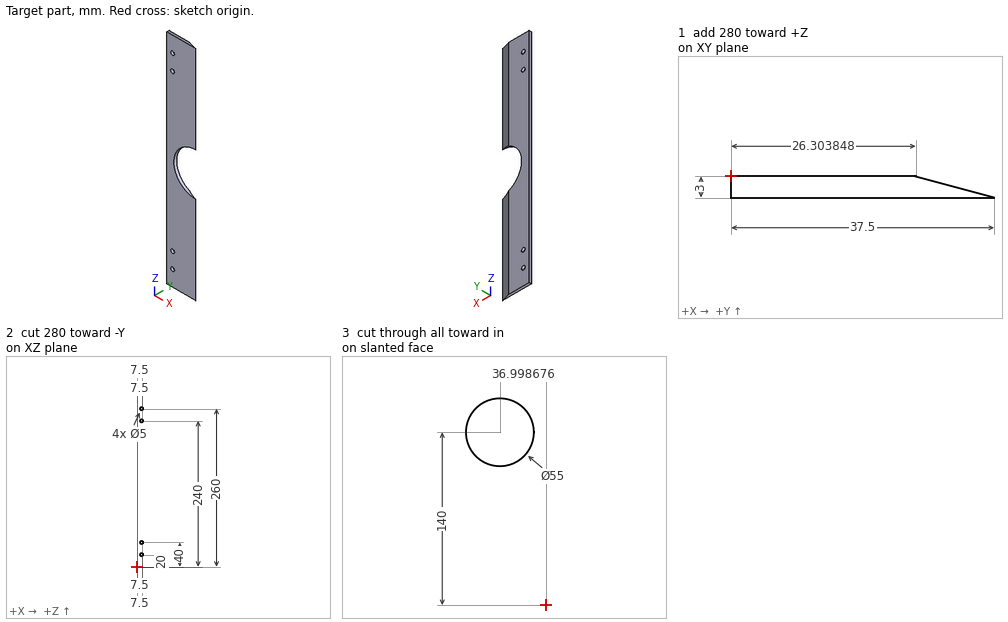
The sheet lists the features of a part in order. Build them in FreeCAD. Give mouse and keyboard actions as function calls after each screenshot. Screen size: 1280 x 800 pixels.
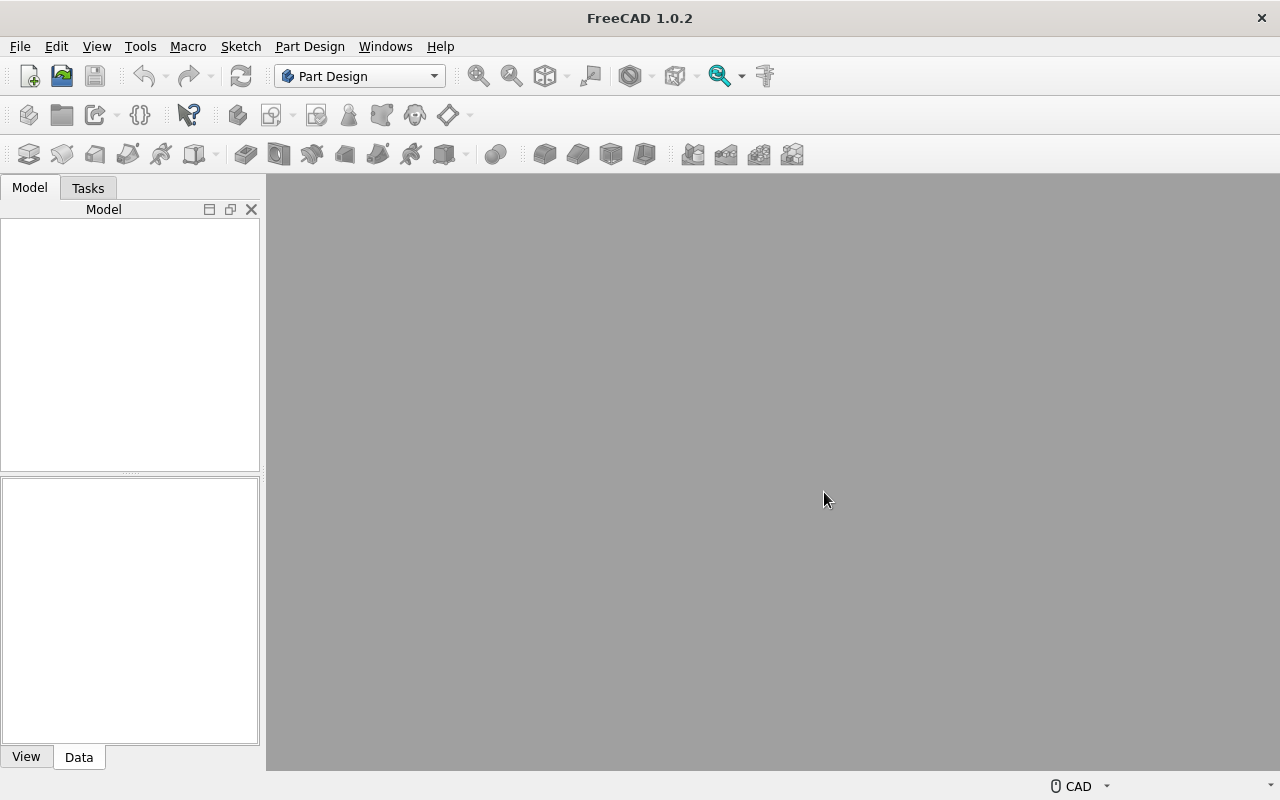
click(29, 76)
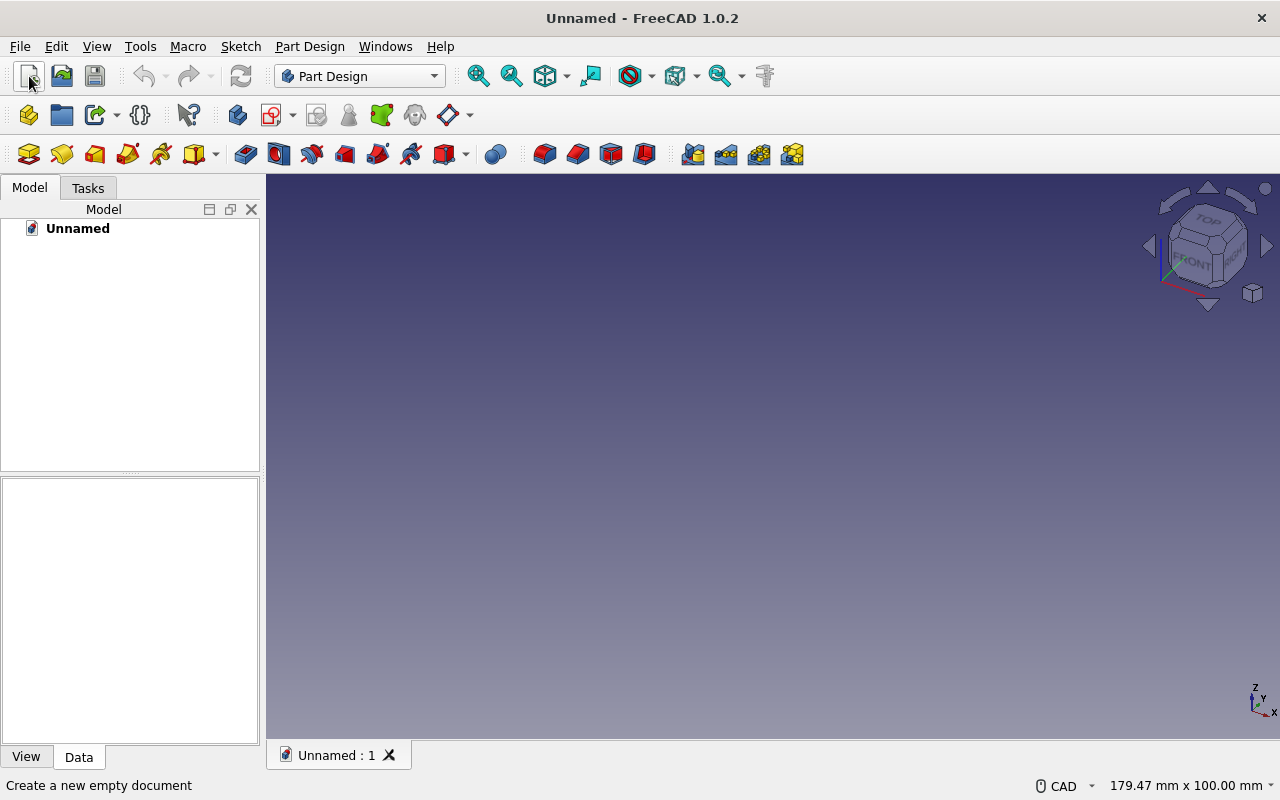
click(270, 116)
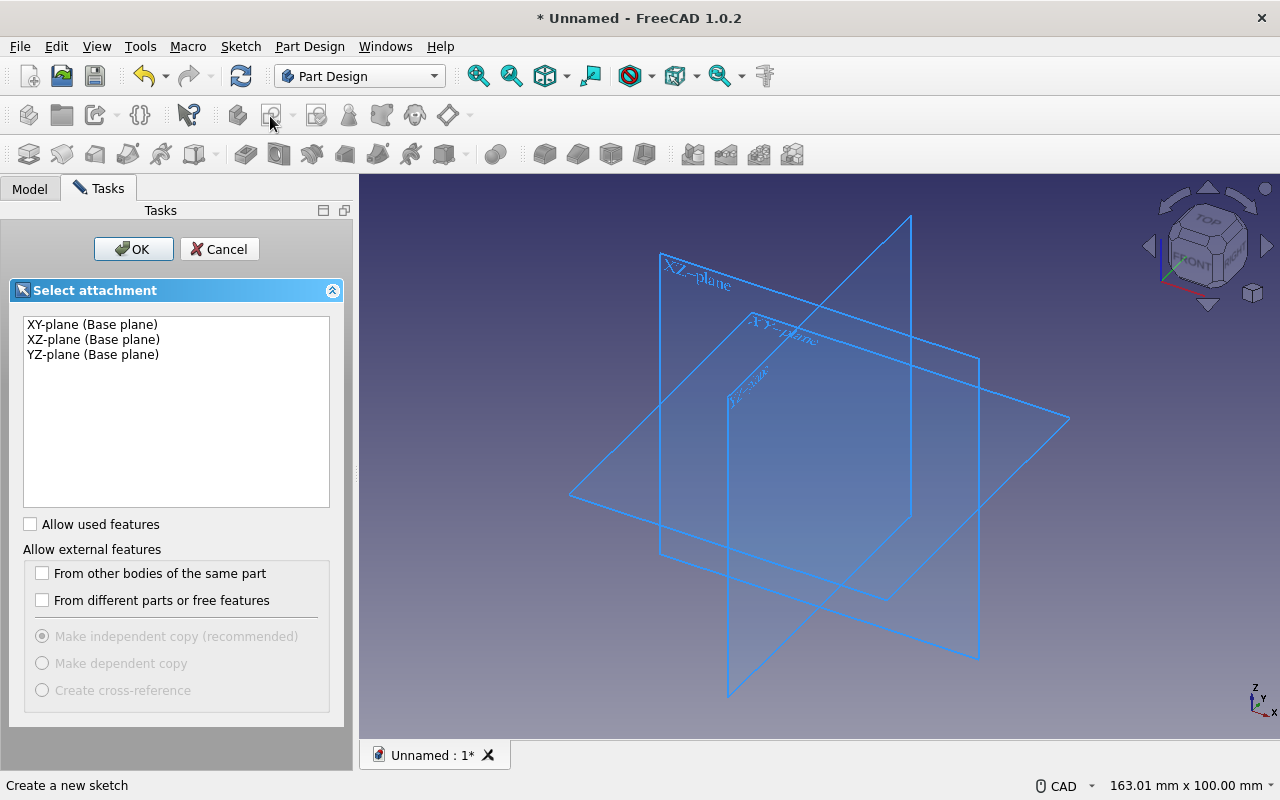
click(84, 324)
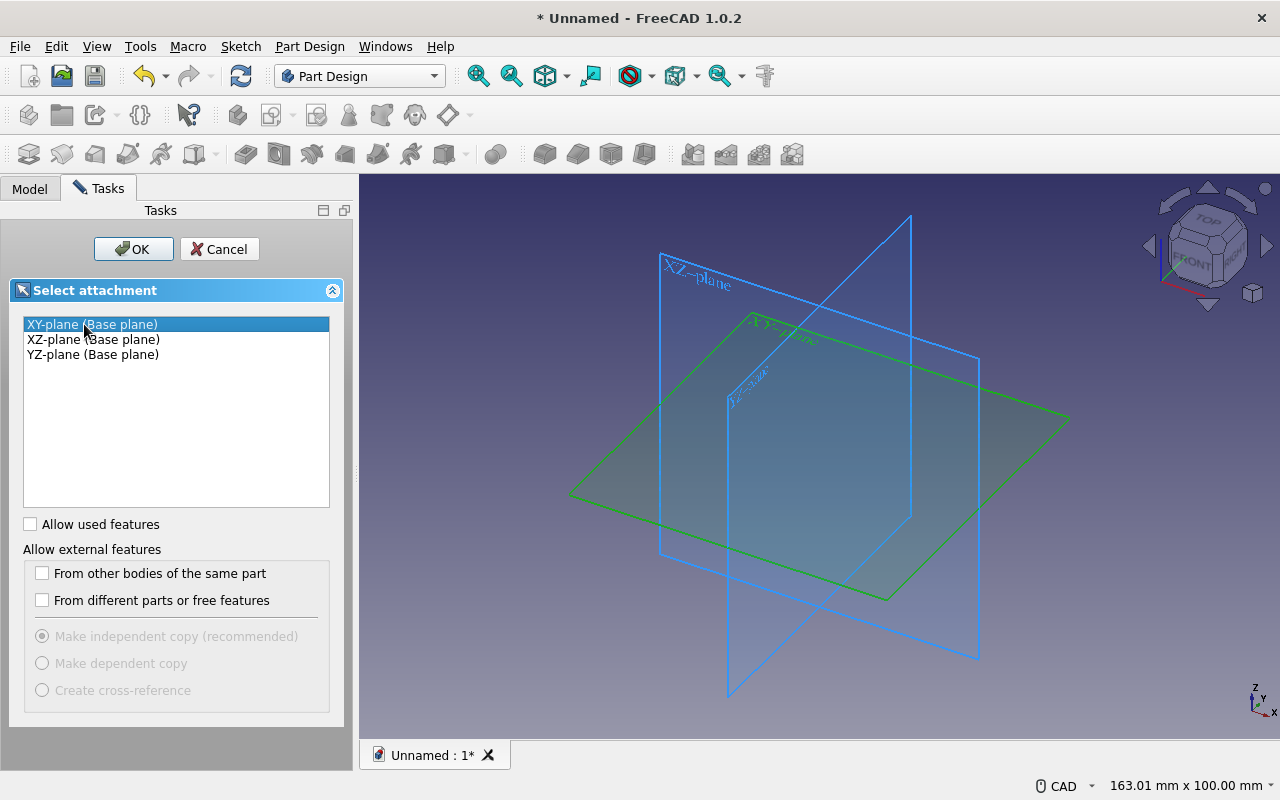
click(134, 249)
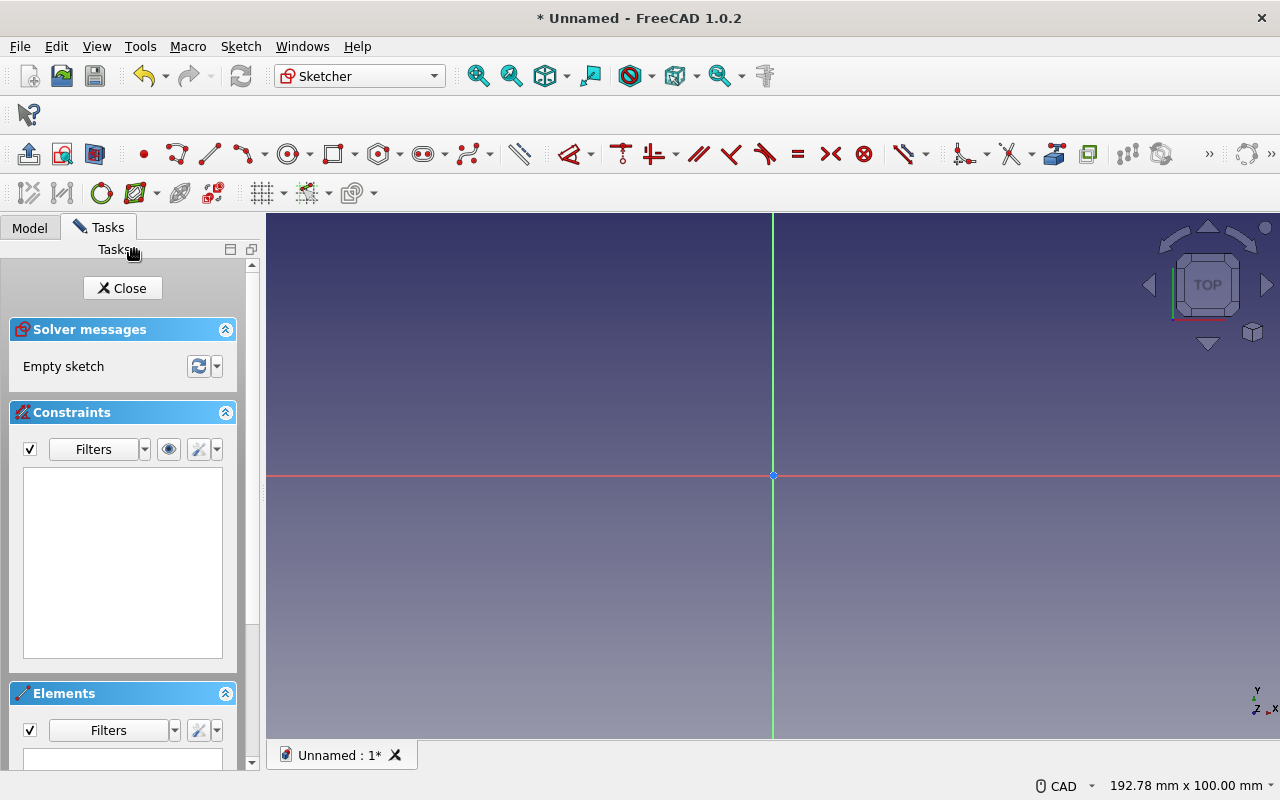
scroll(969, 488, up, 5)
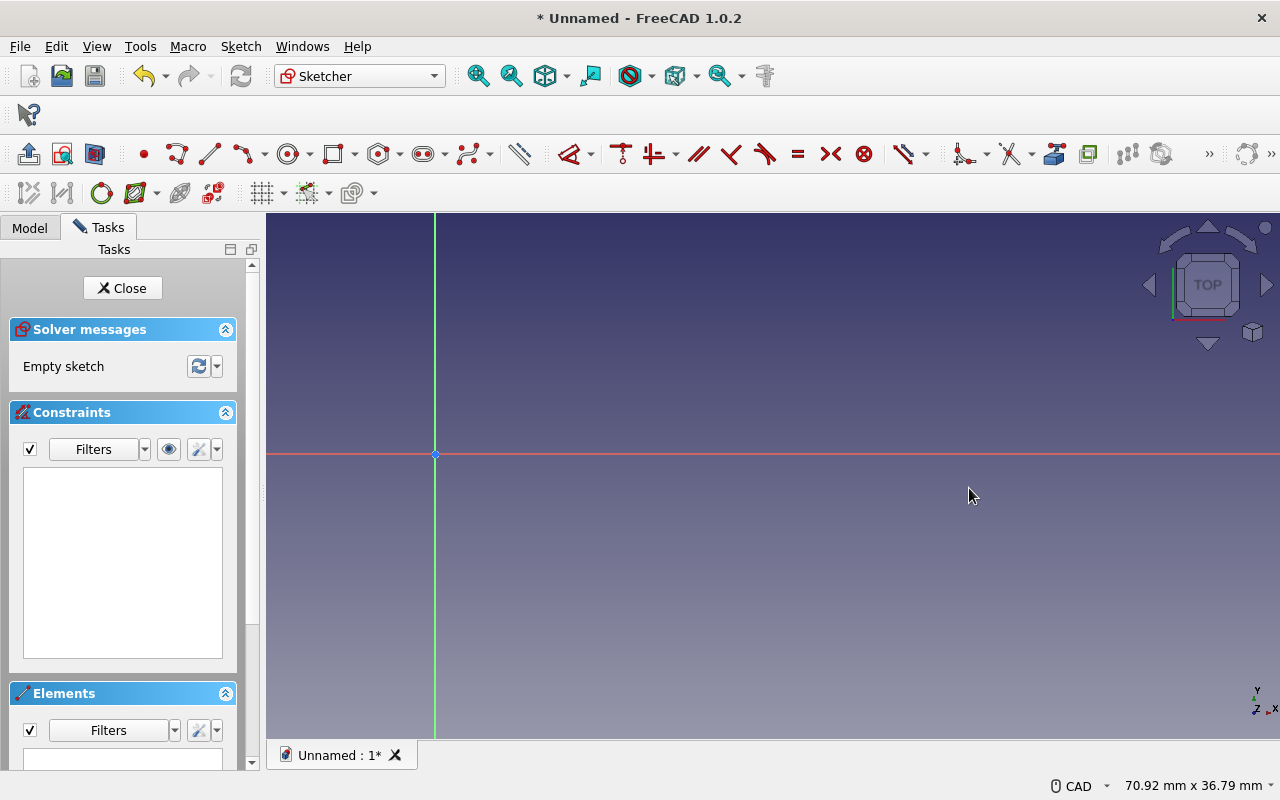
click(177, 154)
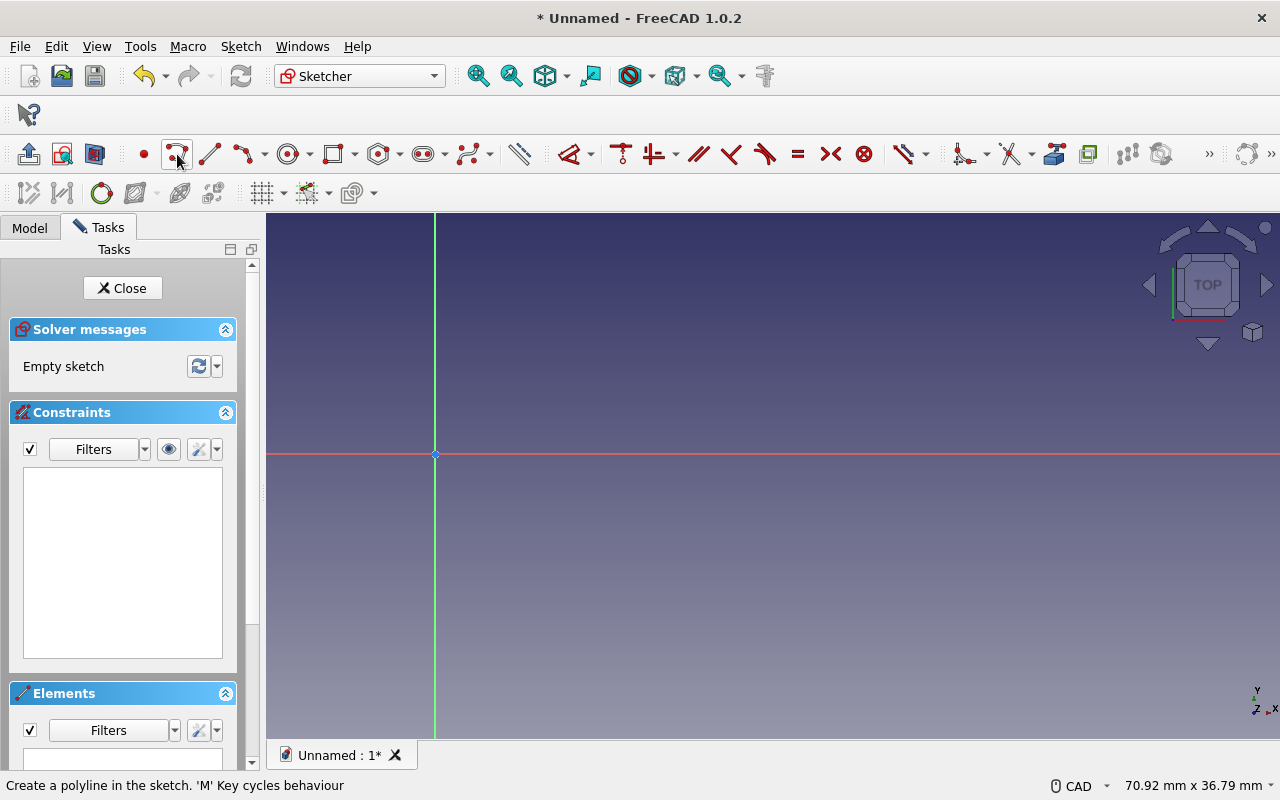
click(435, 454)
click(444, 497)
click(971, 497)
click(811, 463)
click(435, 454)
key(Escape)
key(Escape)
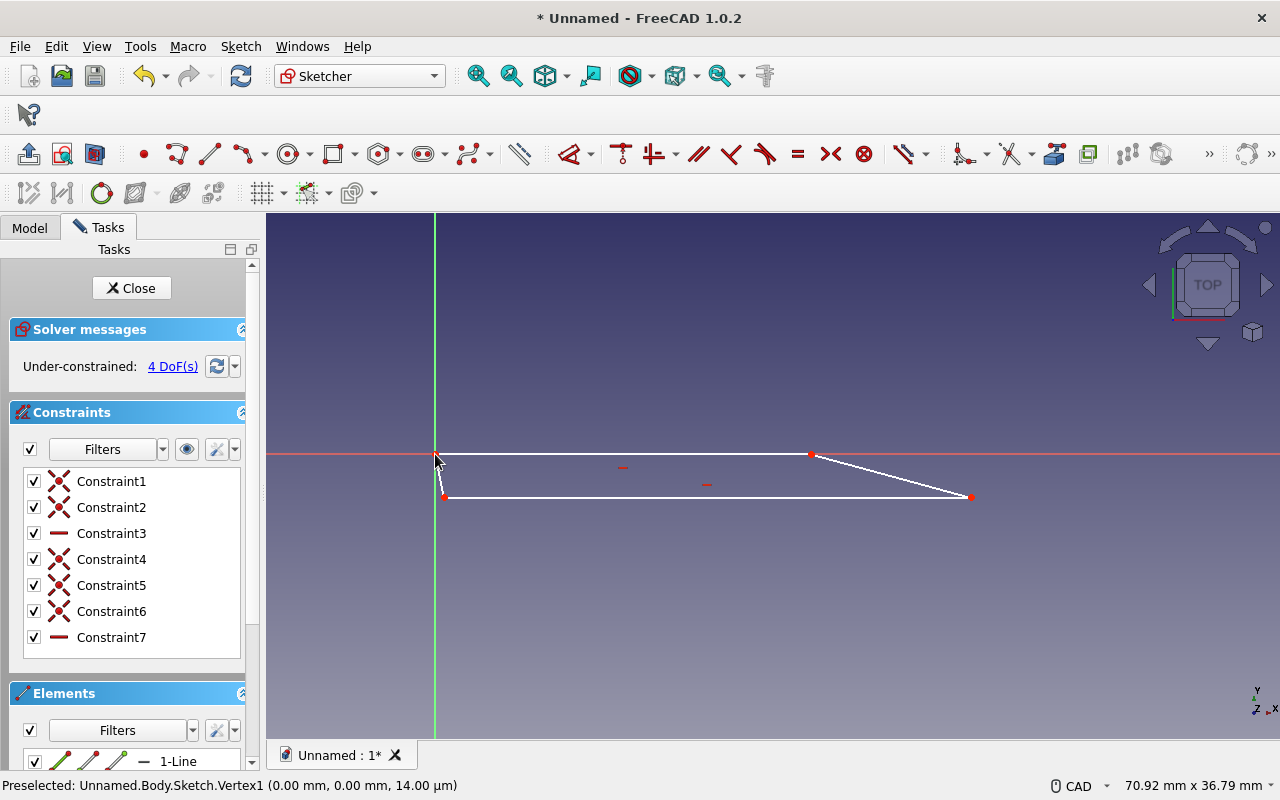
click(438, 468)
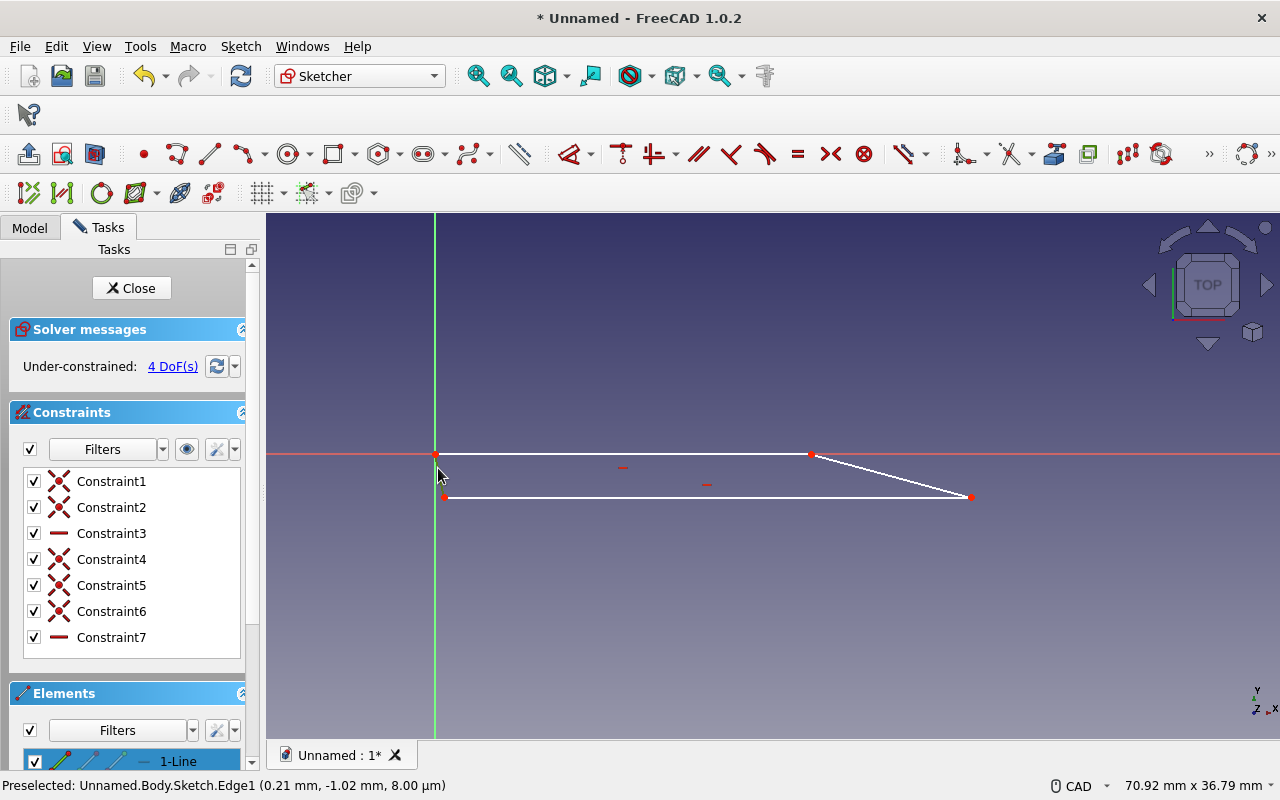
key(v)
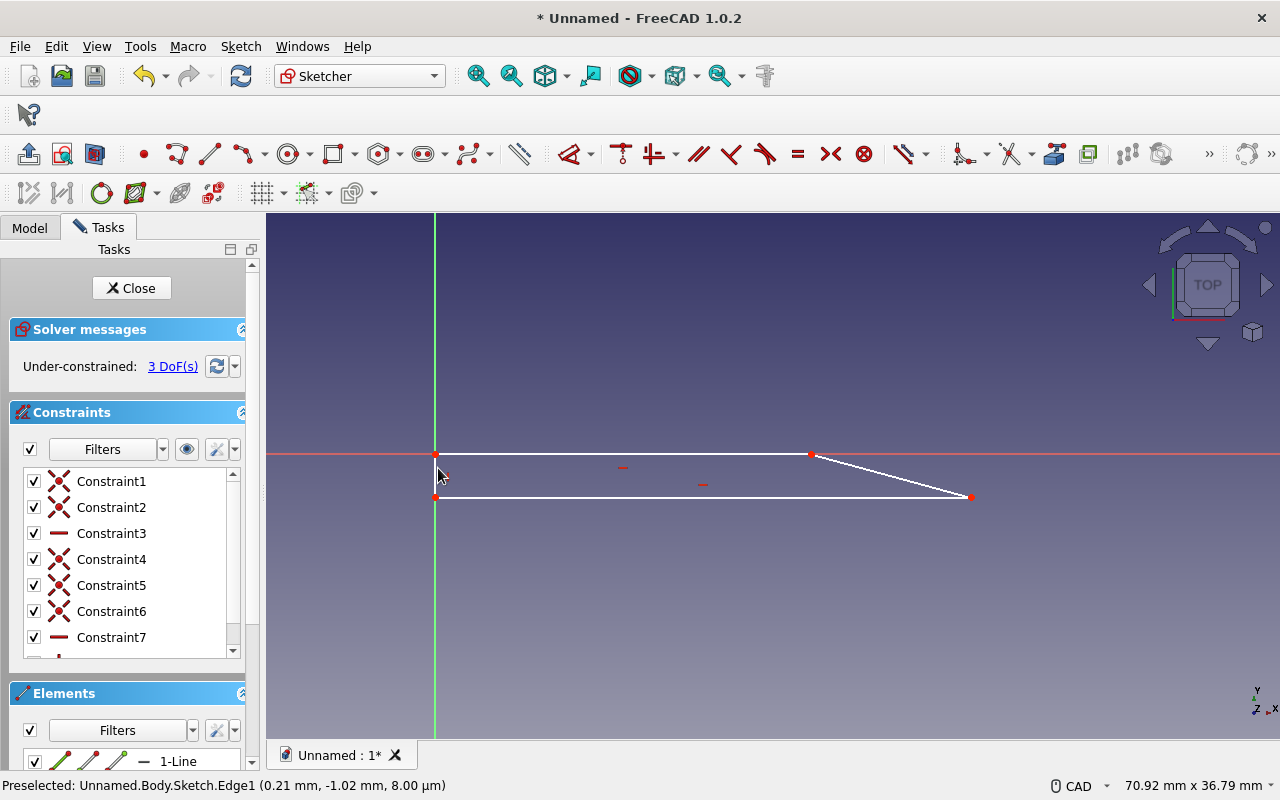
click(568, 154)